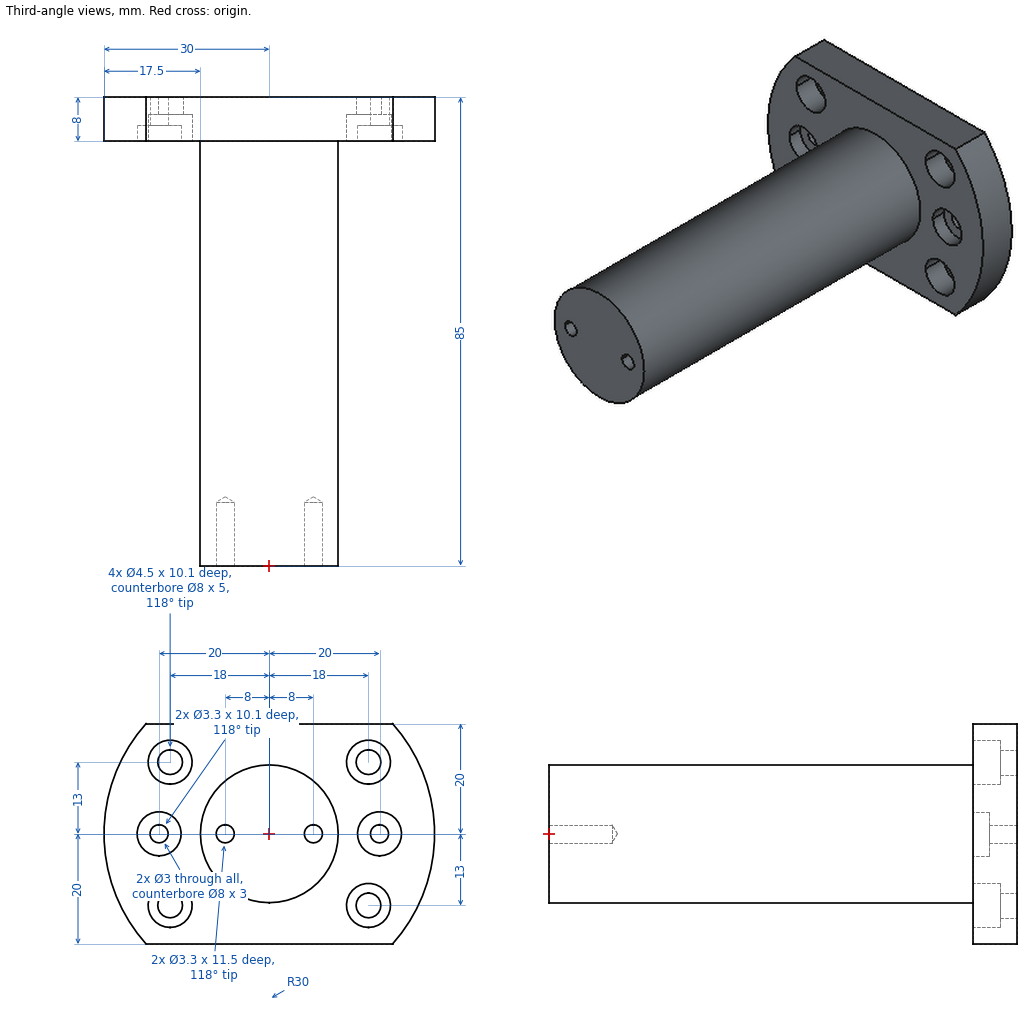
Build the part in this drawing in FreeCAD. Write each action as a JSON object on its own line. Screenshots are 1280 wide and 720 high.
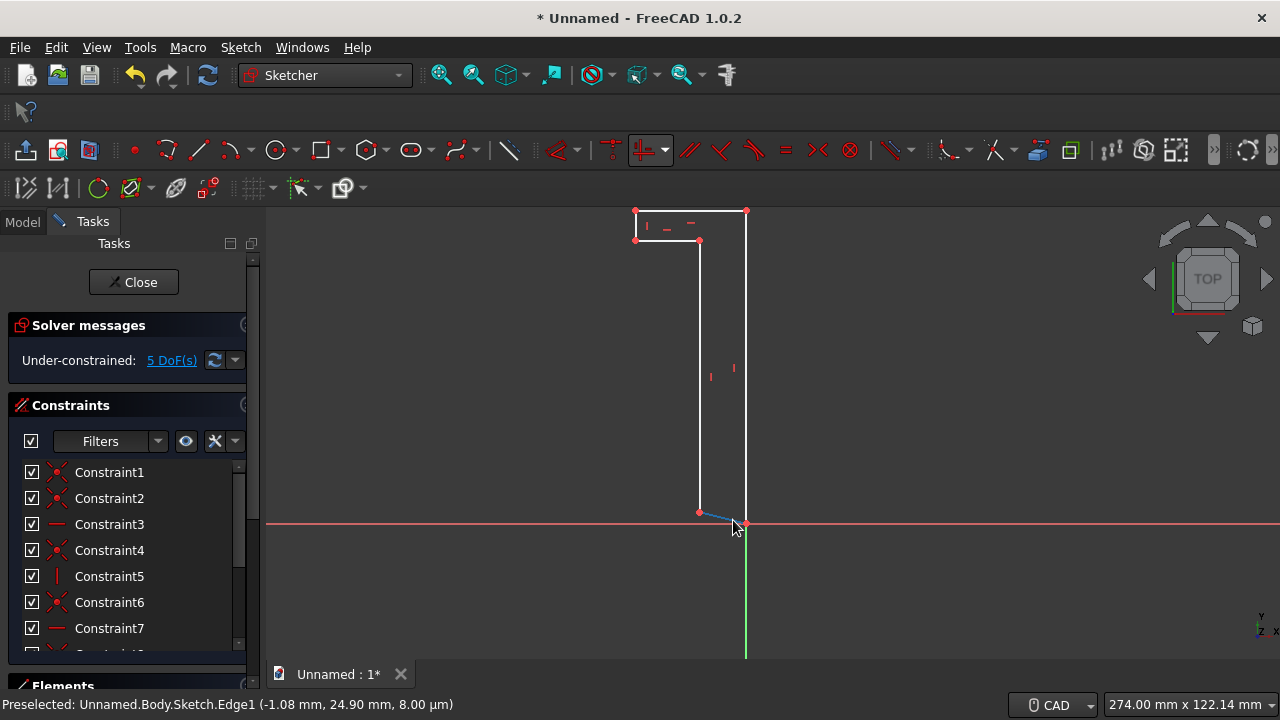
{"action": "left_click", "coordinate": [732, 520]}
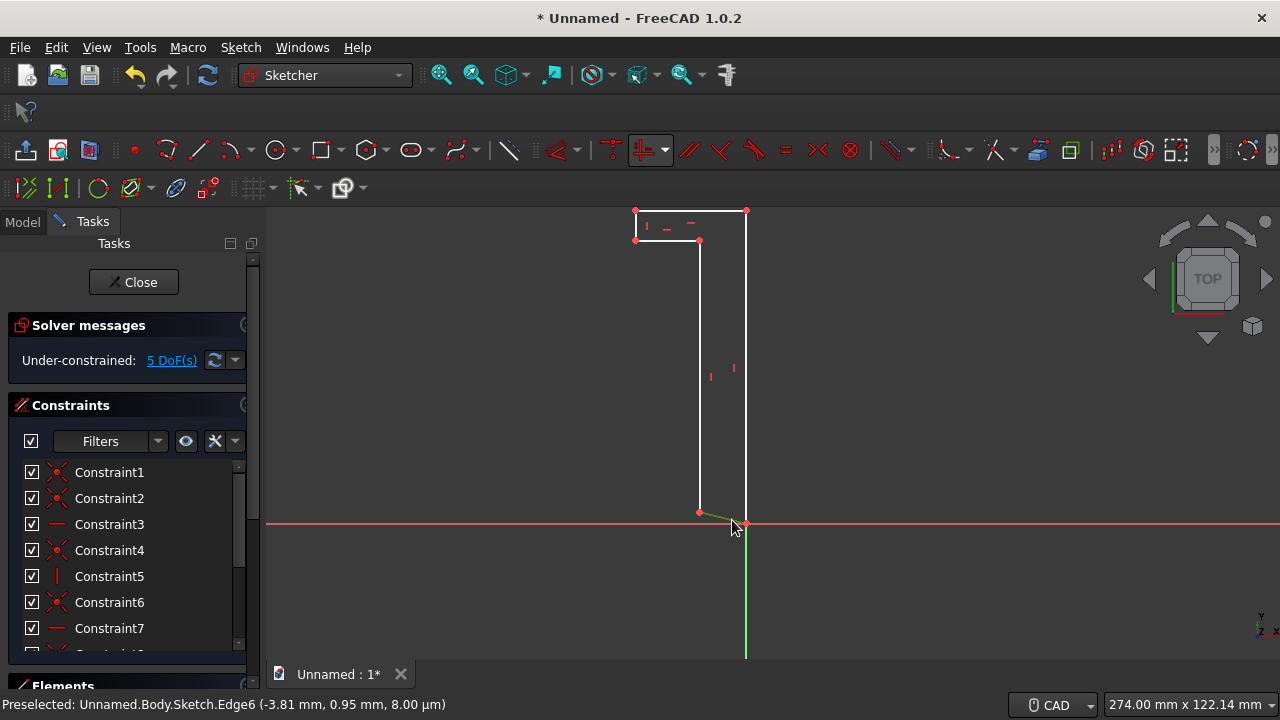
{"action": "left_click", "coordinate": [668, 150]}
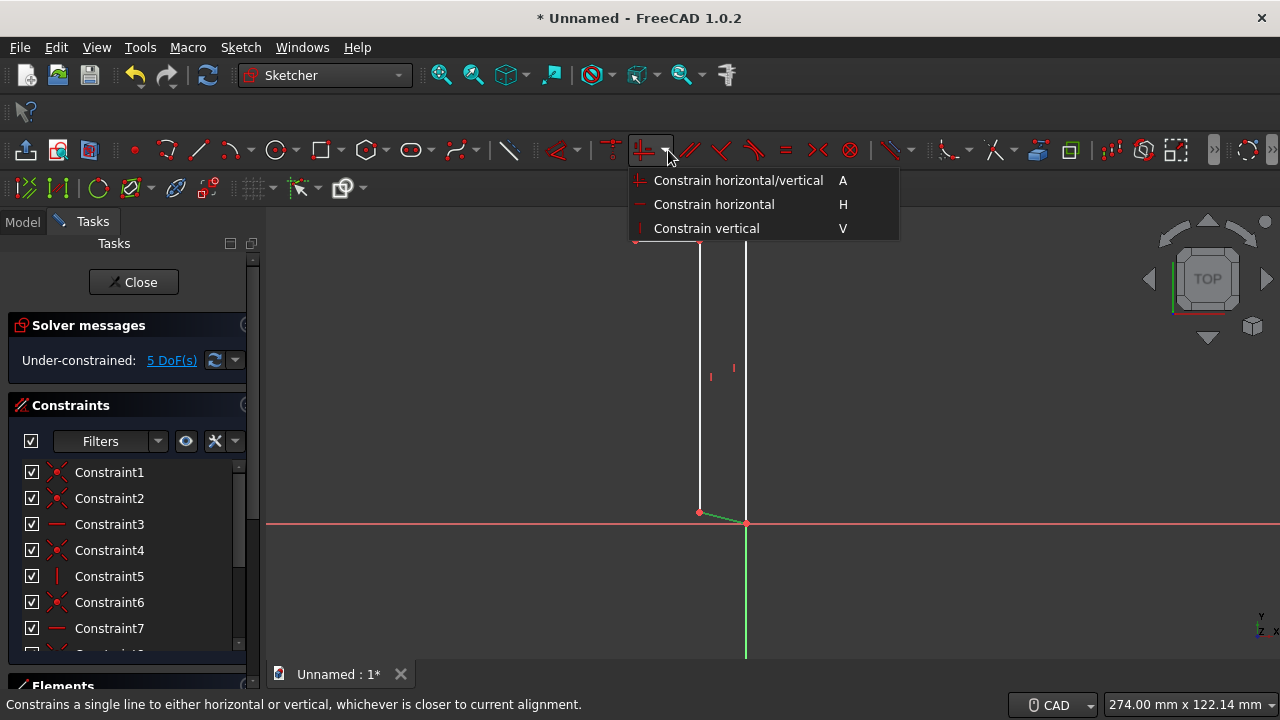
{"action": "left_click", "coordinate": [764, 204]}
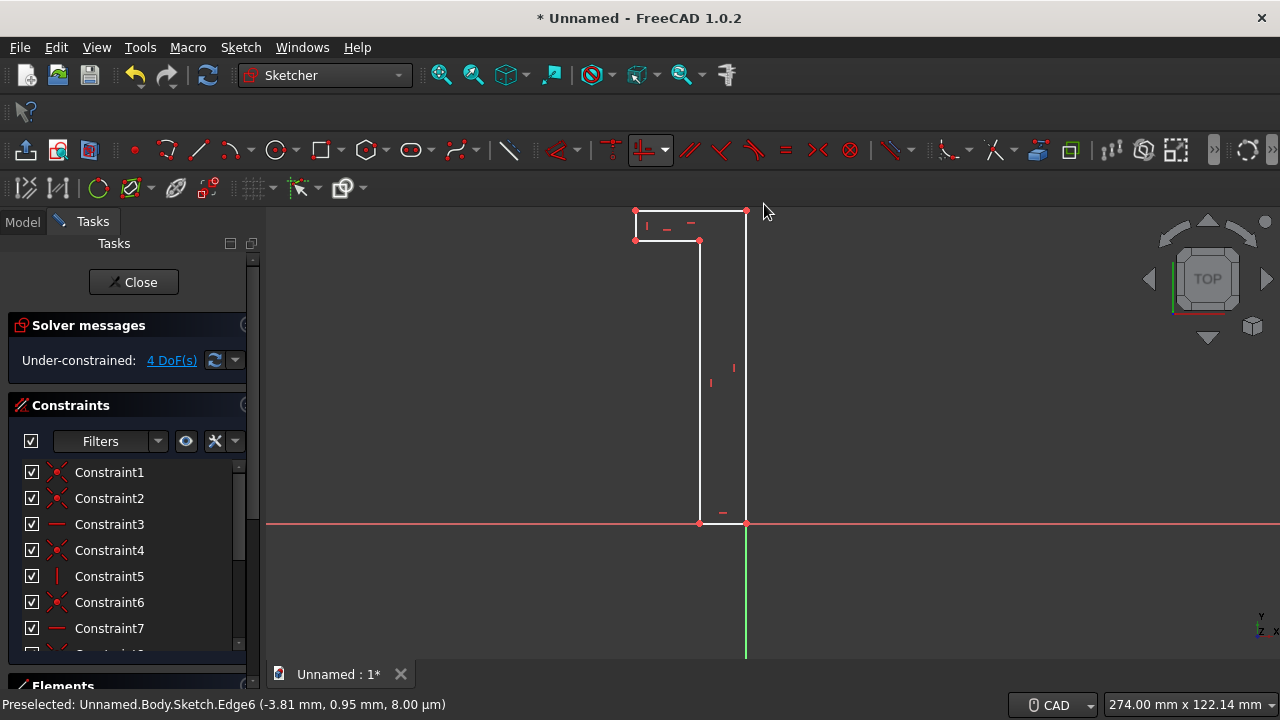
{"action": "left_click", "coordinate": [556, 150]}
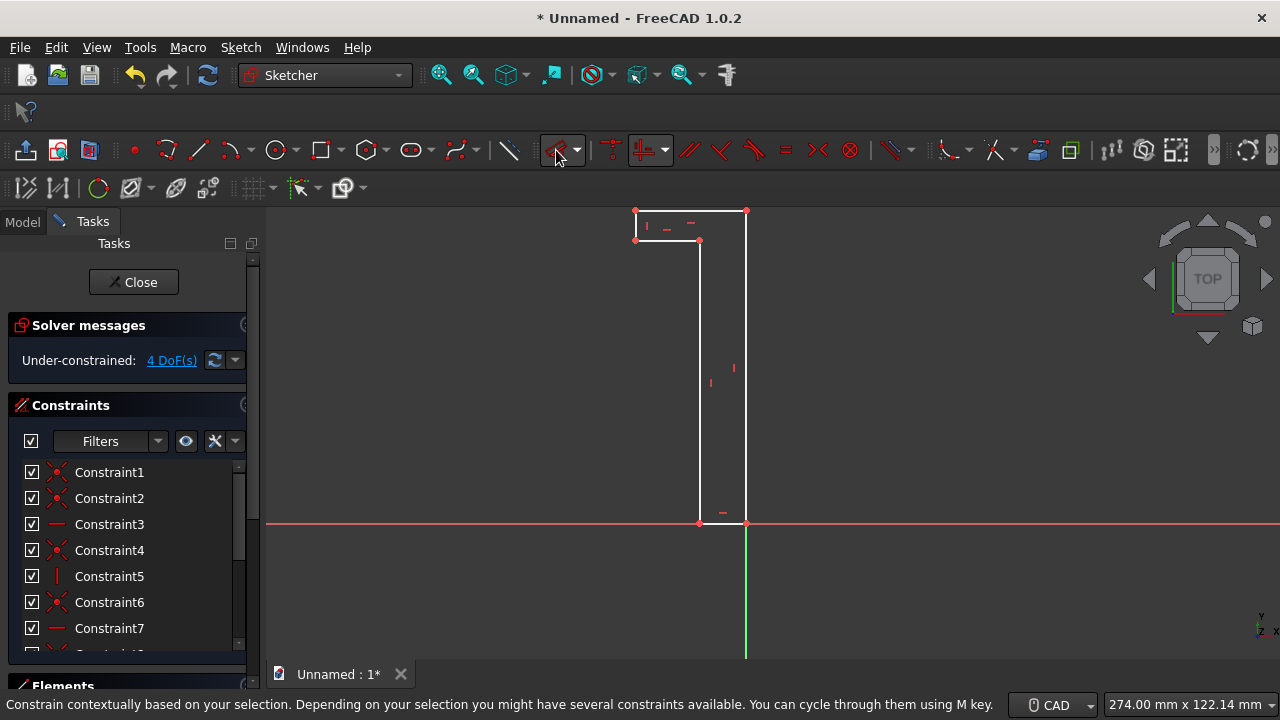
{"action": "scroll", "coordinate": [766, 631], "scroll_direction": "down", "scroll_amount": 1}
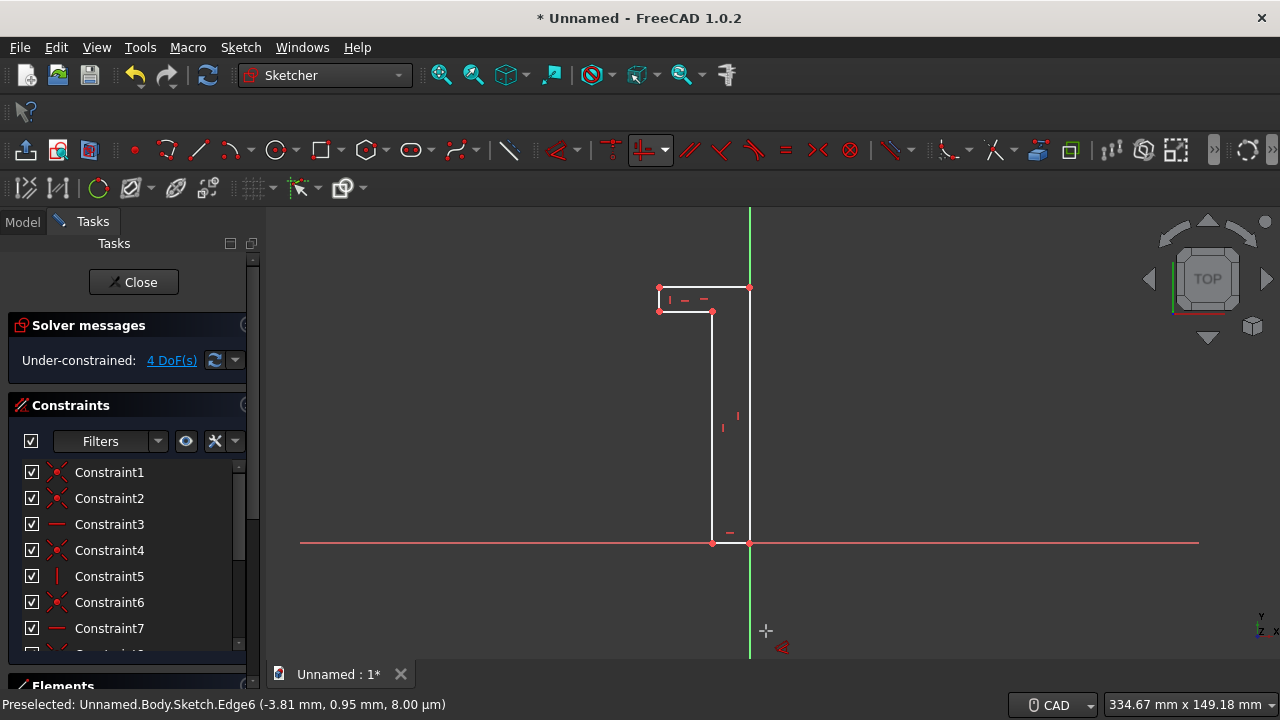
{"action": "scroll", "coordinate": [659, 297], "scroll_direction": "up", "scroll_amount": 3}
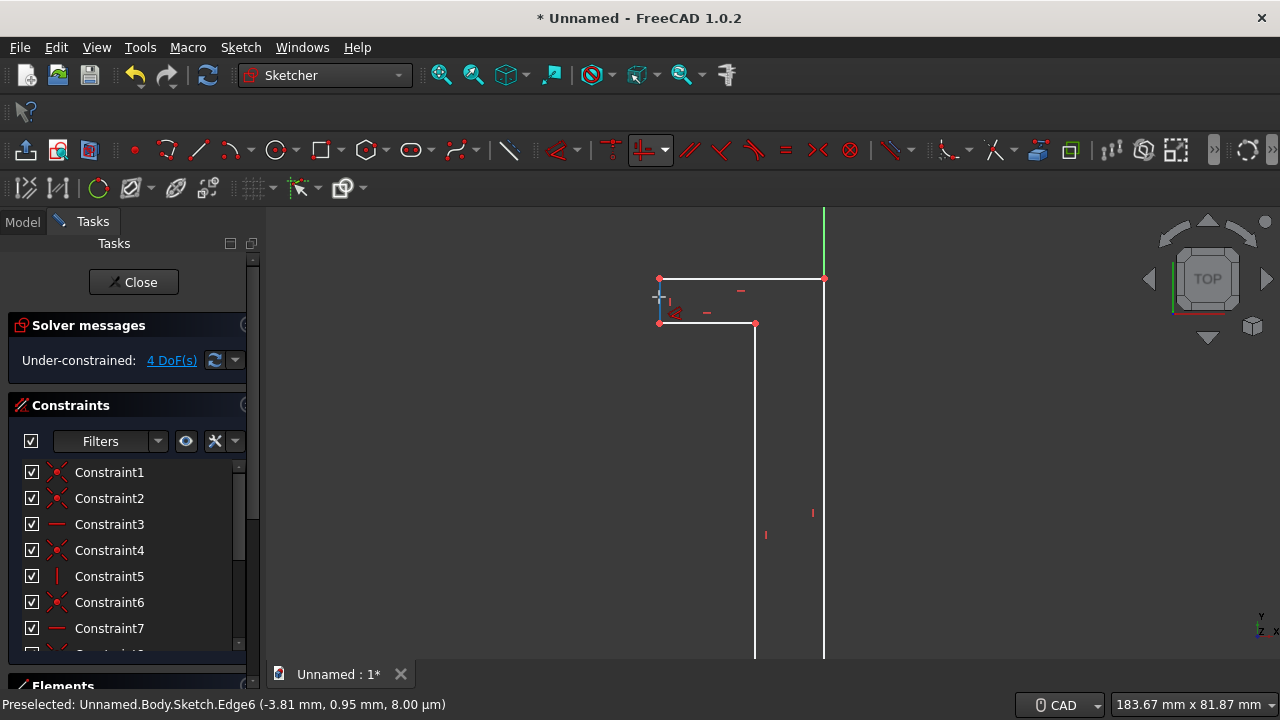
{"action": "left_click", "coordinate": [660, 297]}
{"action": "left_click", "coordinate": [626, 301]}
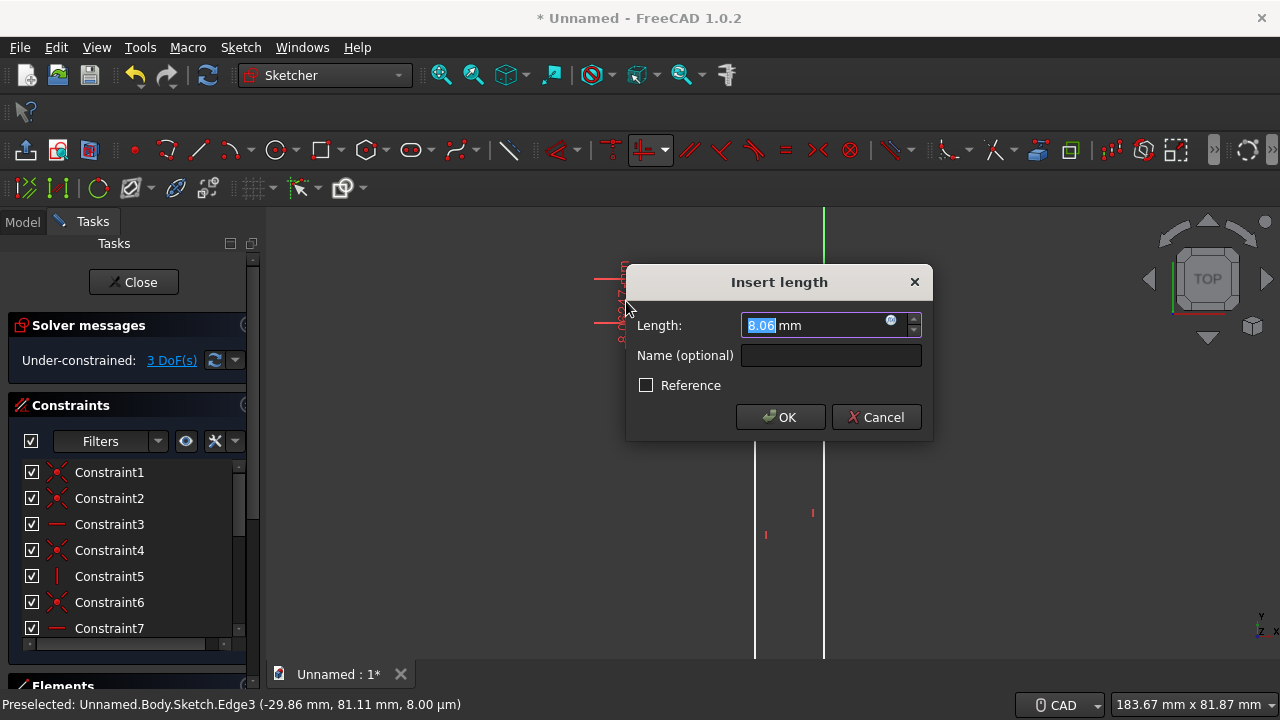
{"action": "type", "text": "8"}
{"action": "key", "text": "Return"}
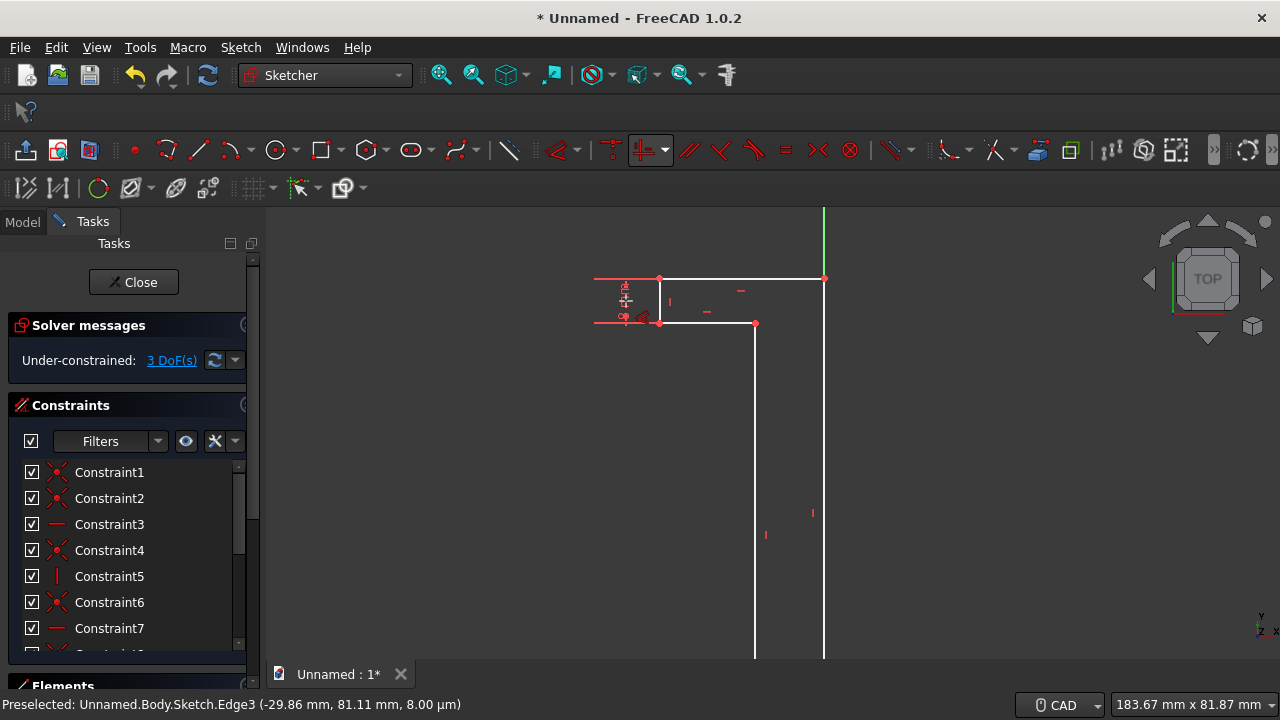
{"action": "left_click", "coordinate": [824, 606]}
{"action": "left_click", "coordinate": [858, 455]}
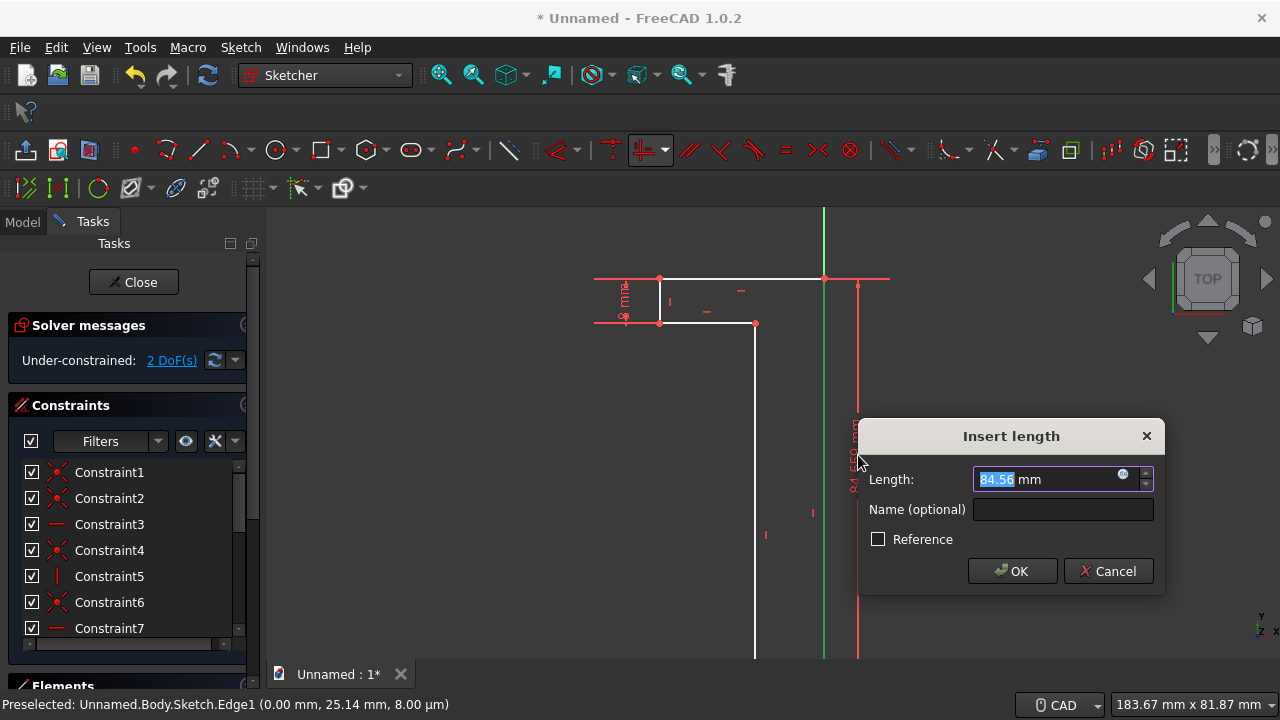
{"action": "type", "text": "85"}
{"action": "key", "text": "Return"}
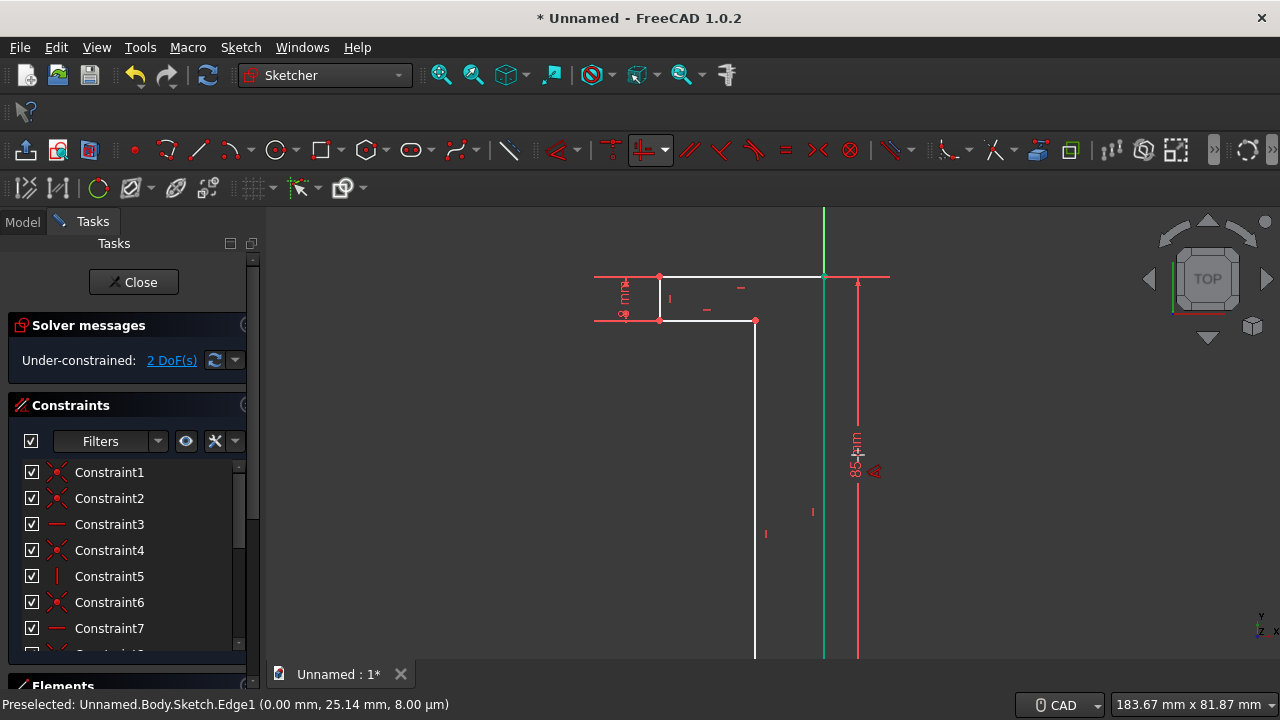
{"action": "left_click", "coordinate": [775, 277]}
{"action": "left_click", "coordinate": [742, 243]}